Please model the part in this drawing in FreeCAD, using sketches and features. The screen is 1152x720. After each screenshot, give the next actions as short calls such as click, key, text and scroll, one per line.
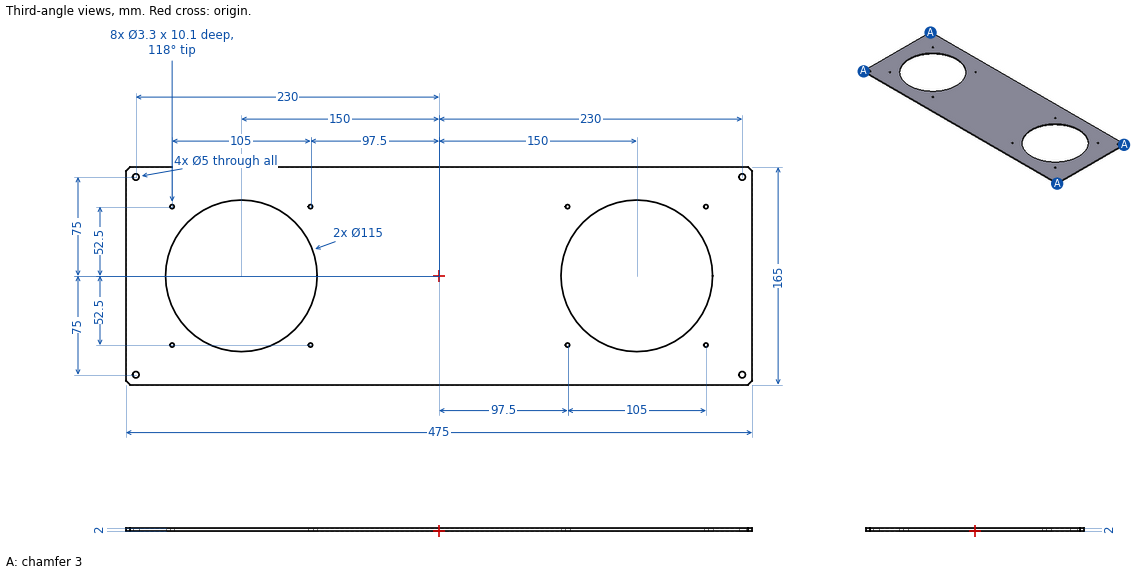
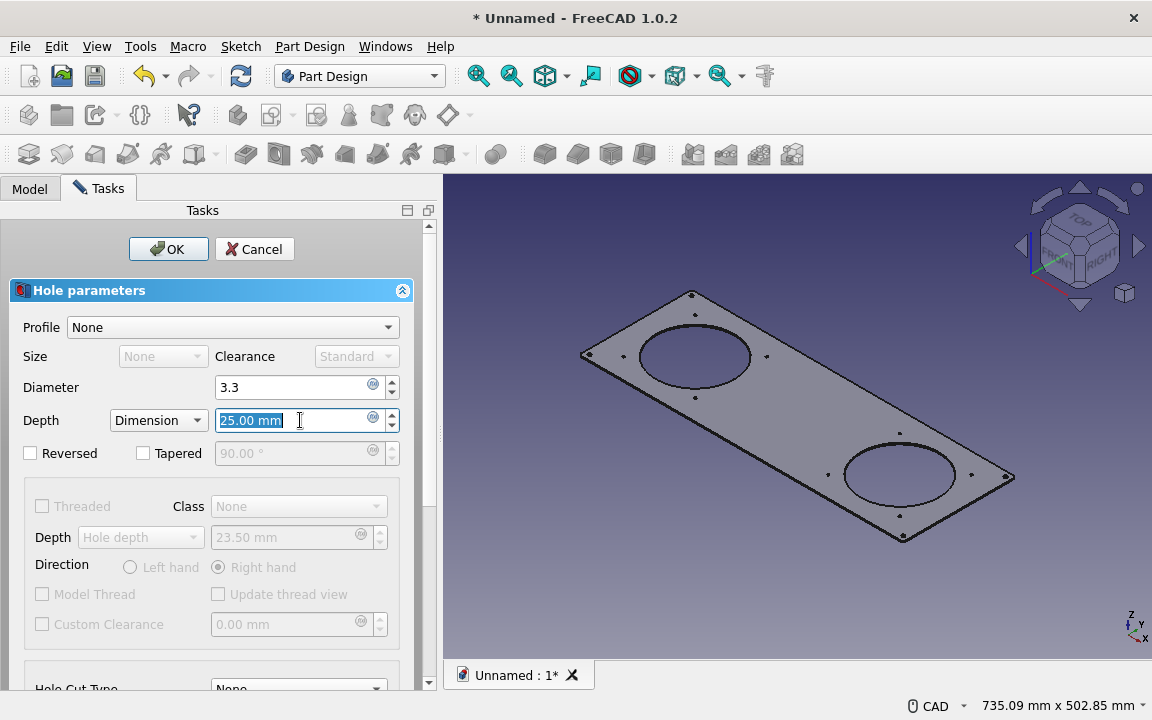
text(10.1)
key(Tab)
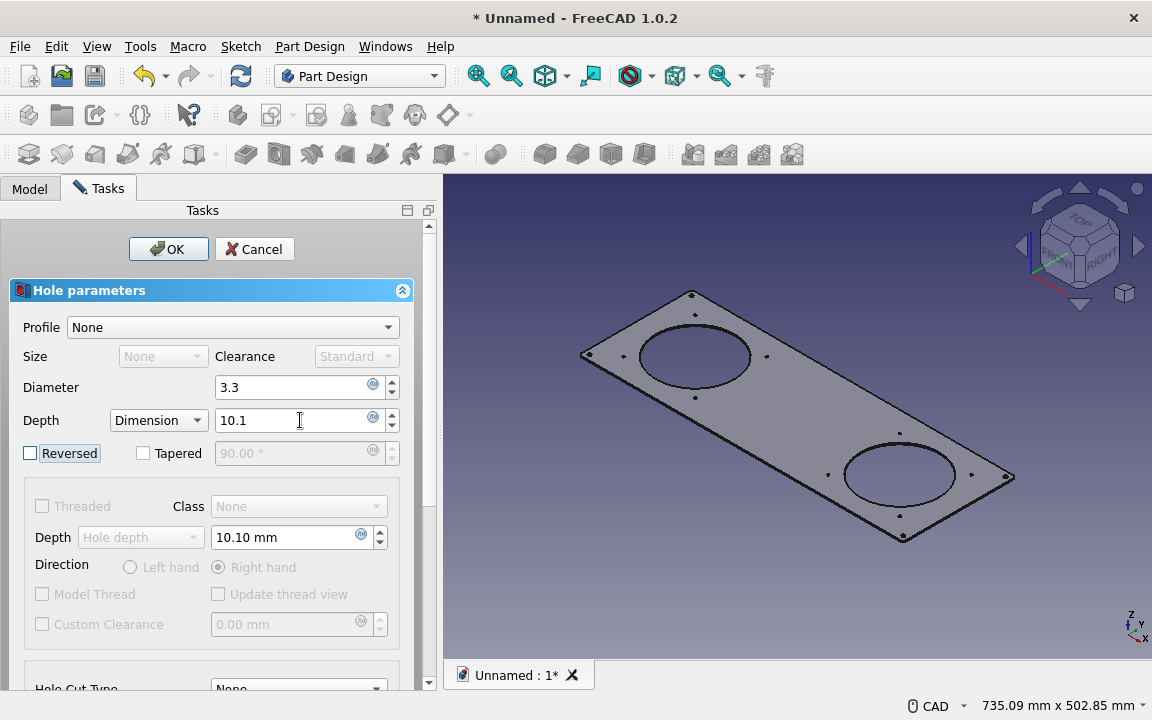
click(169, 249)